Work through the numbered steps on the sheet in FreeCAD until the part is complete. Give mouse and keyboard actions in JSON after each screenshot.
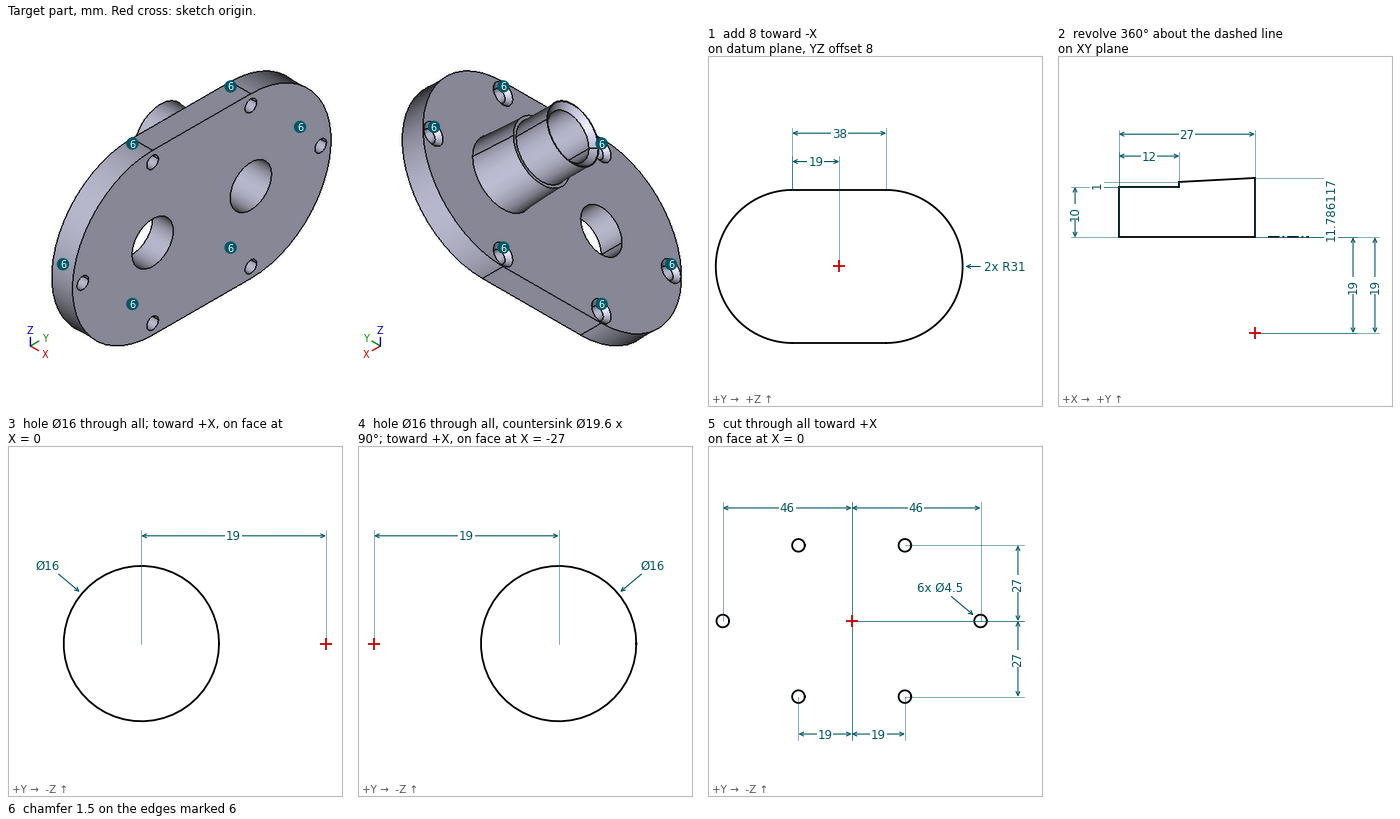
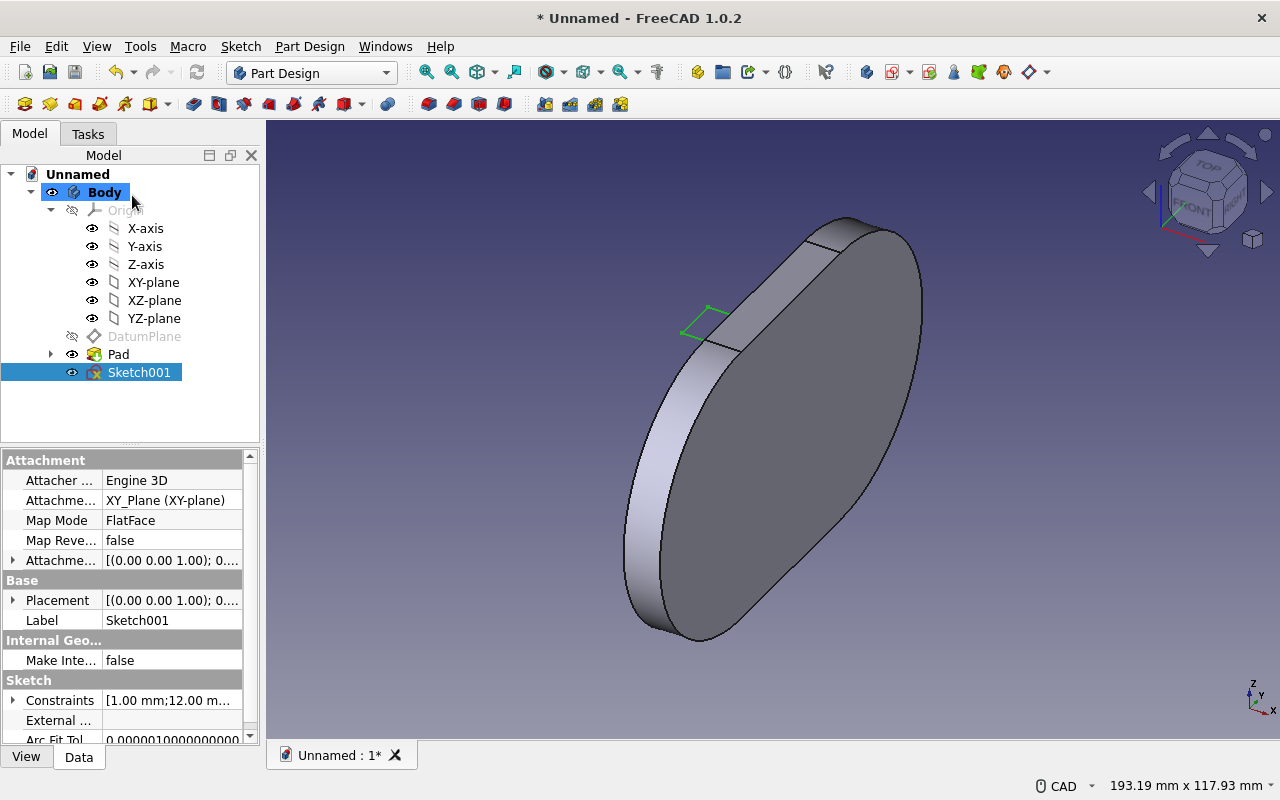
{"action": "left_click", "coordinate": [50, 104]}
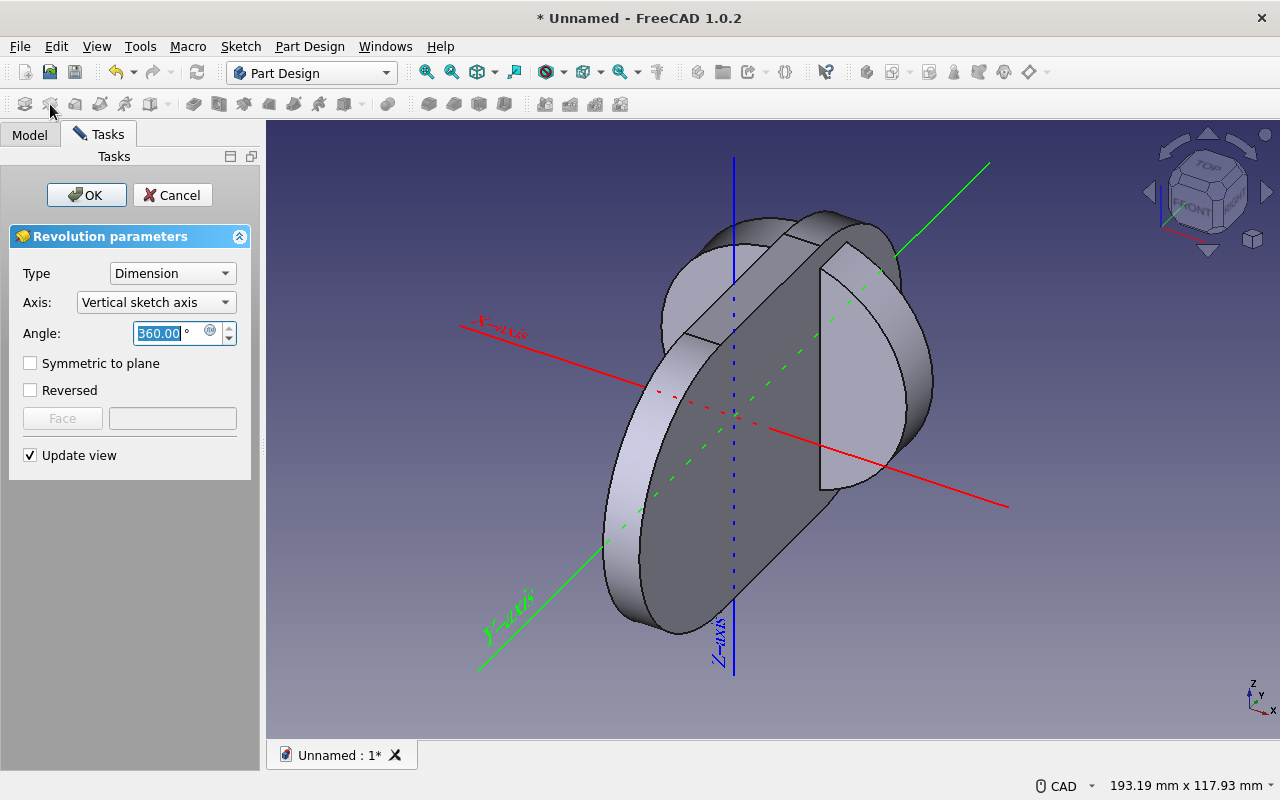
{"action": "left_click", "coordinate": [157, 302]}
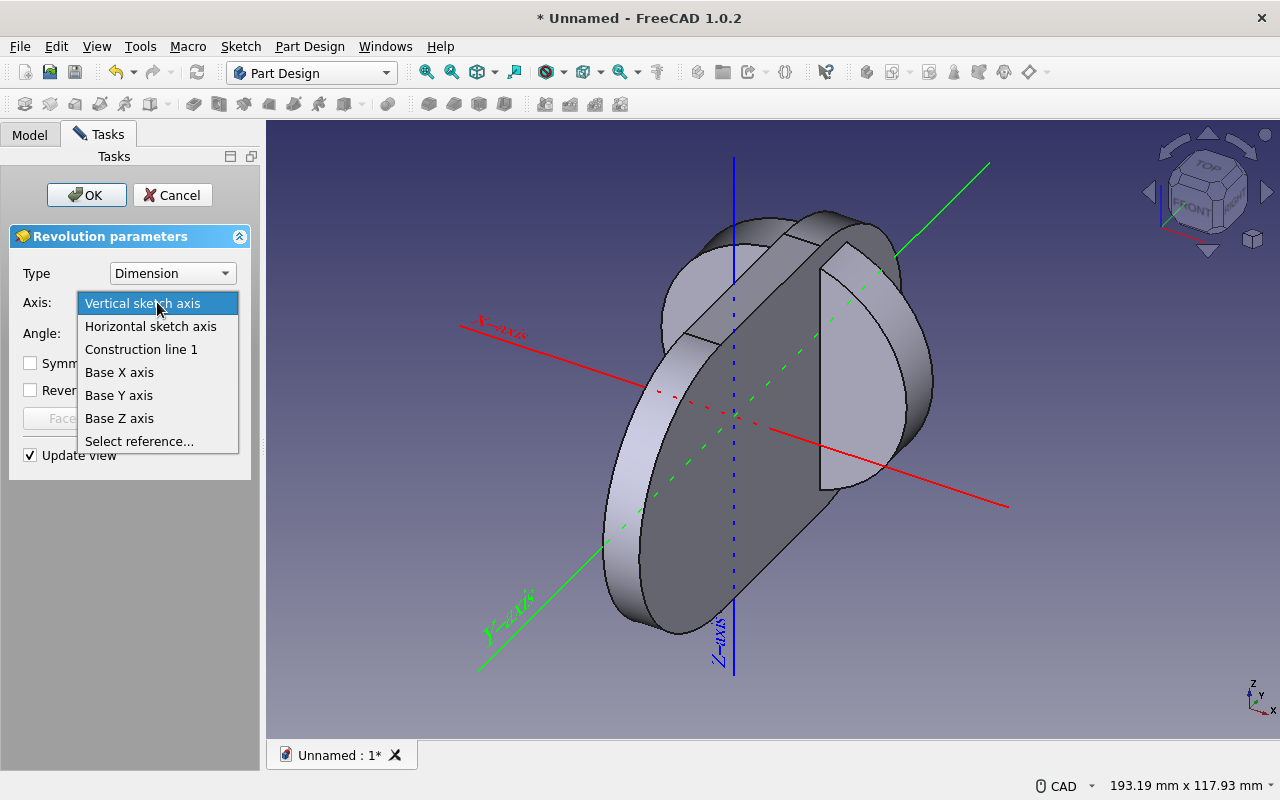
{"action": "left_click", "coordinate": [156, 350]}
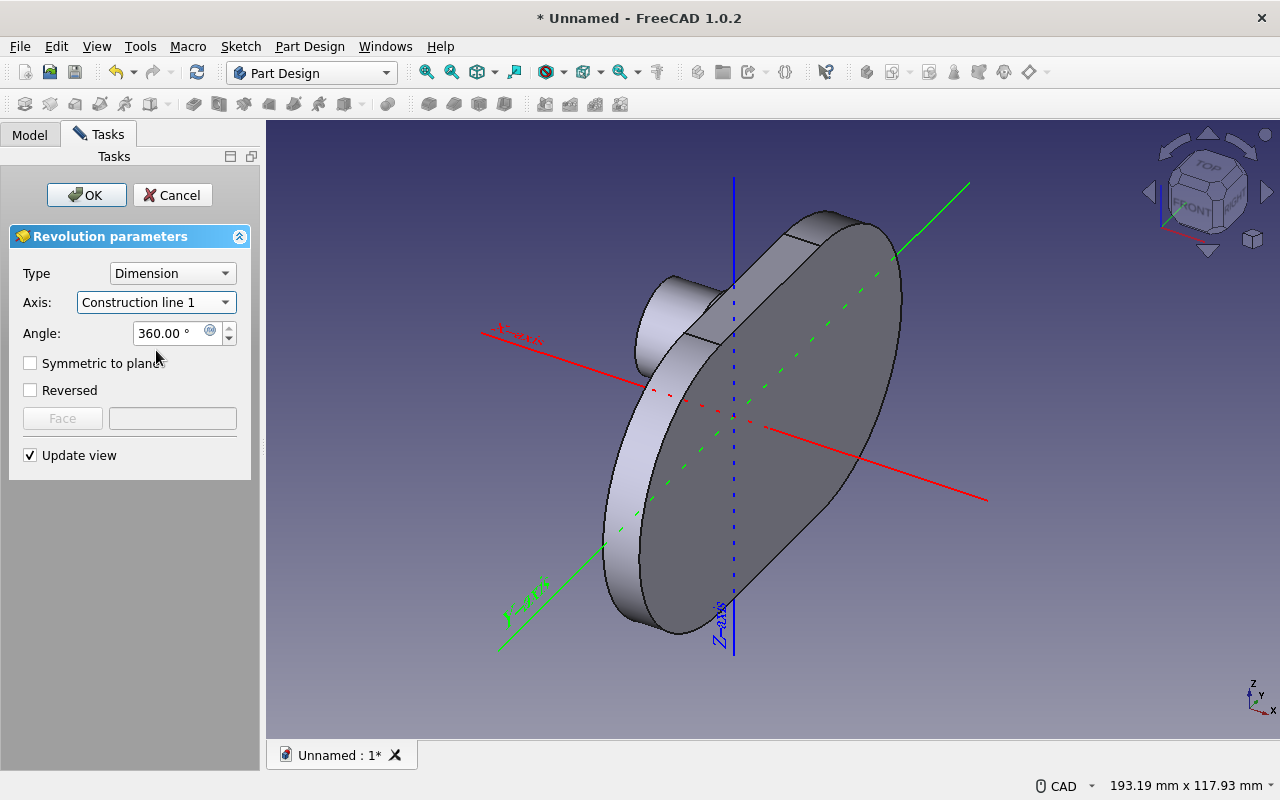
{"action": "left_click", "coordinate": [87, 195]}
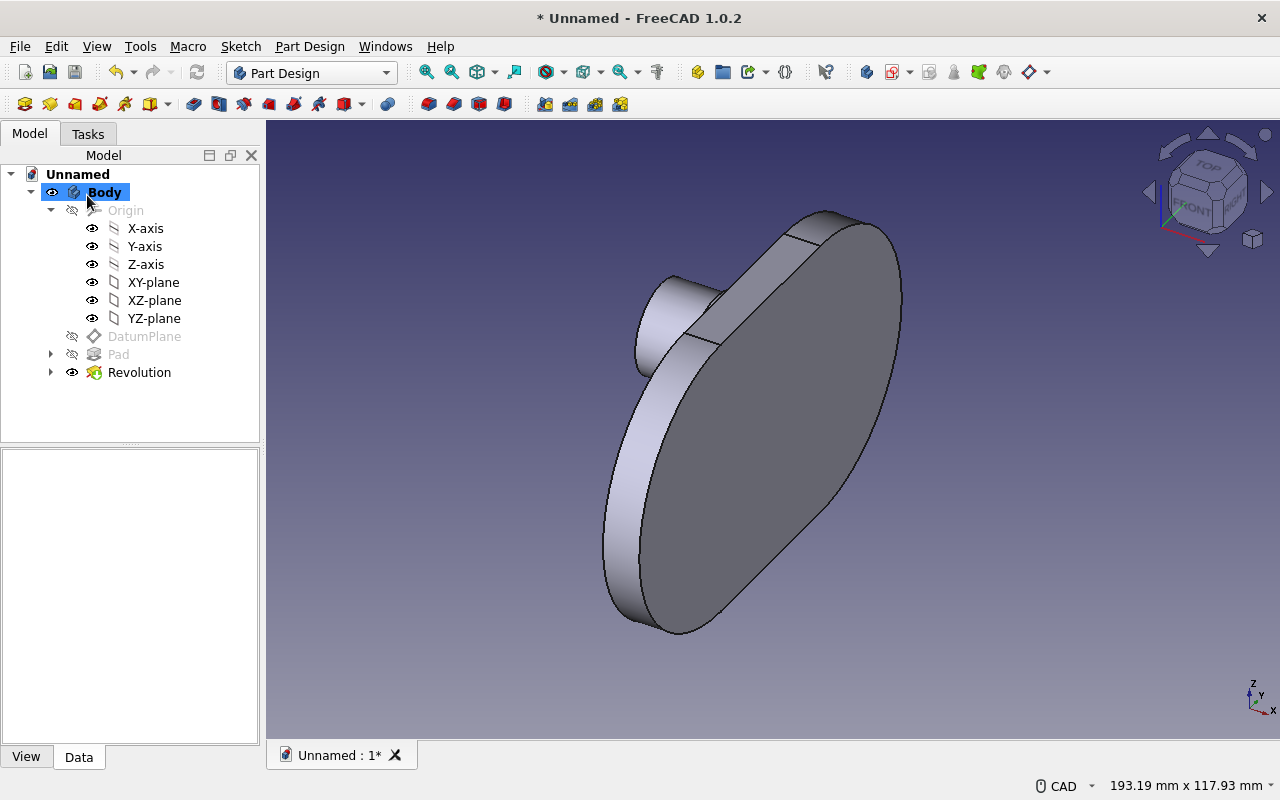
{"action": "left_click", "coordinate": [427, 72]}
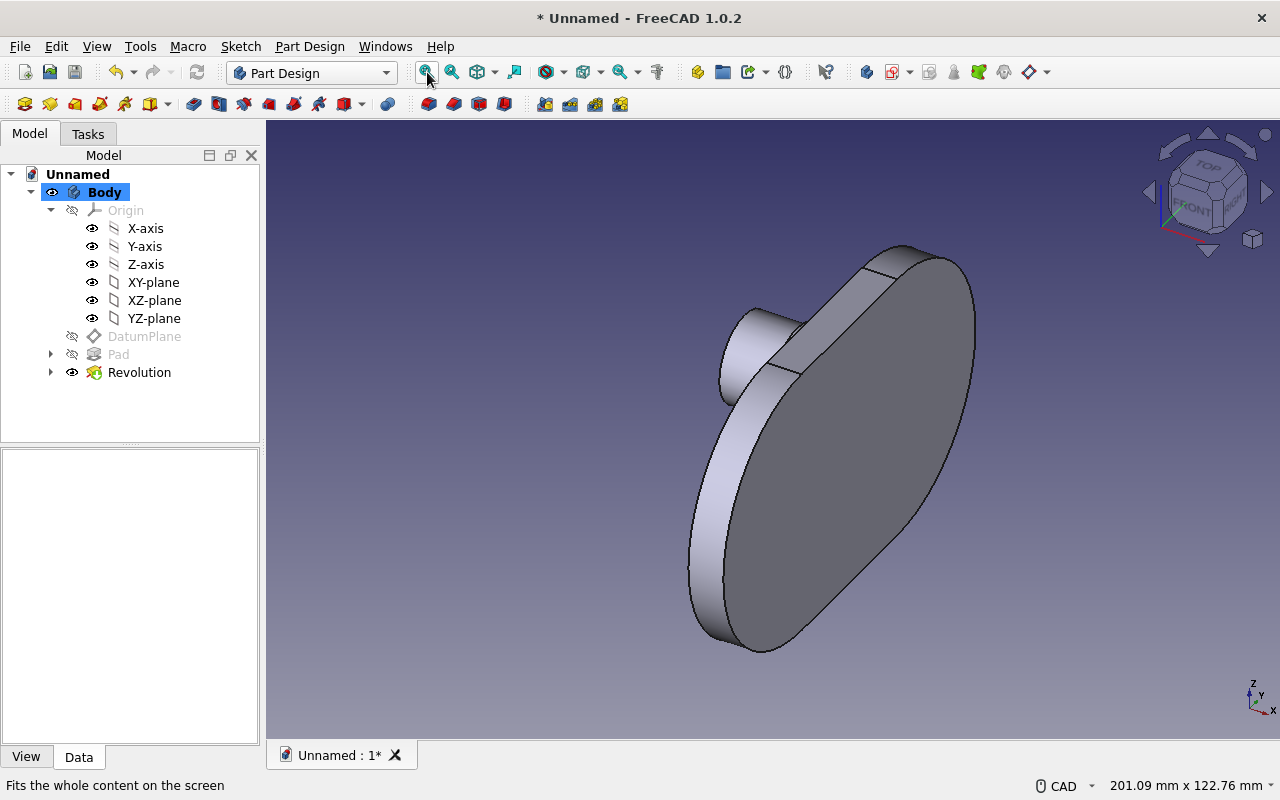
{"action": "key", "text": "6"}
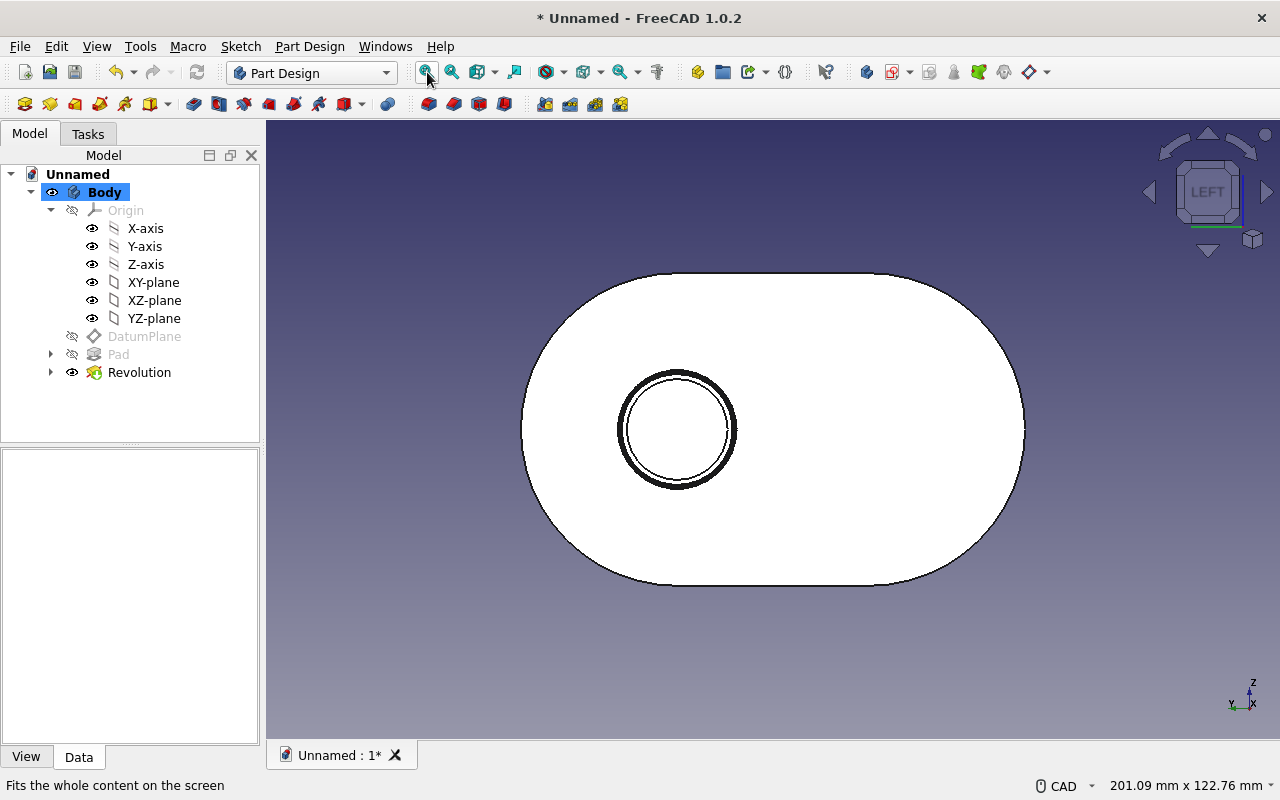
{"action": "left_click", "coordinate": [845, 384]}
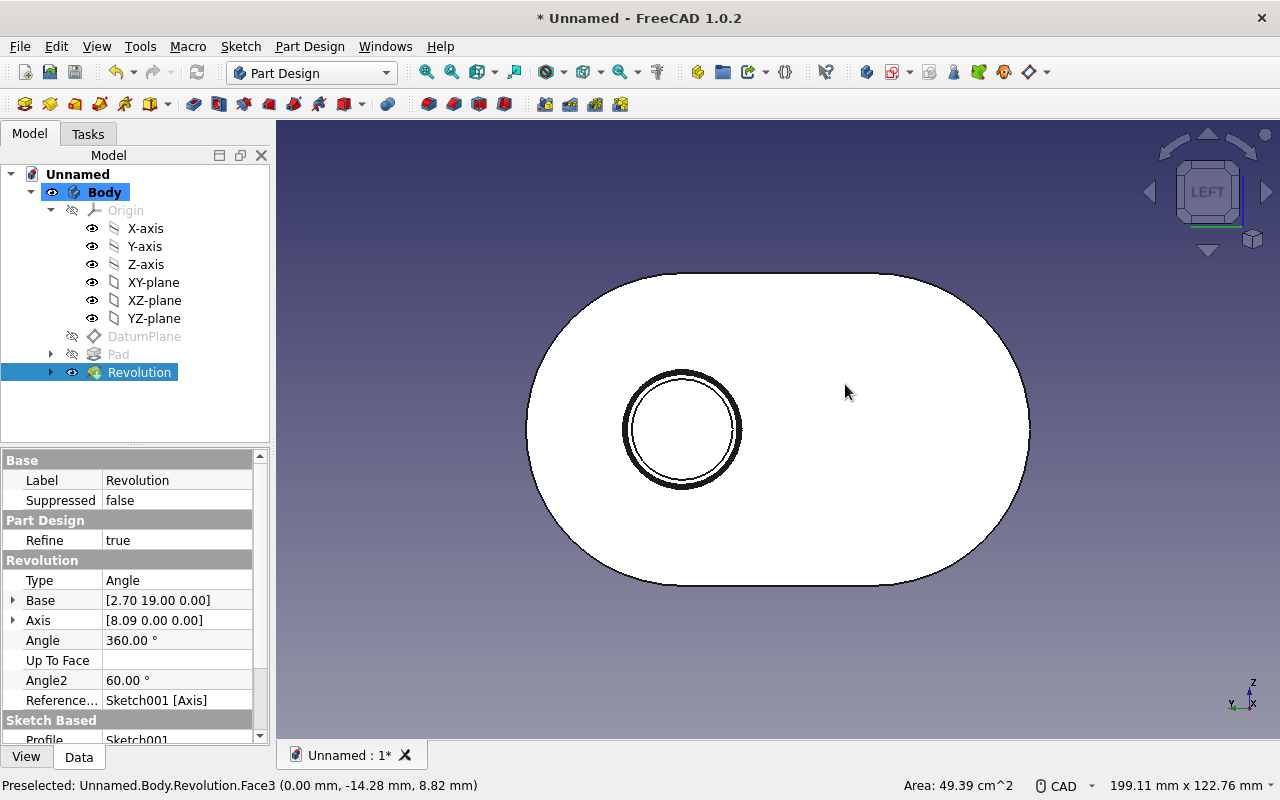
{"action": "left_click", "coordinate": [892, 72]}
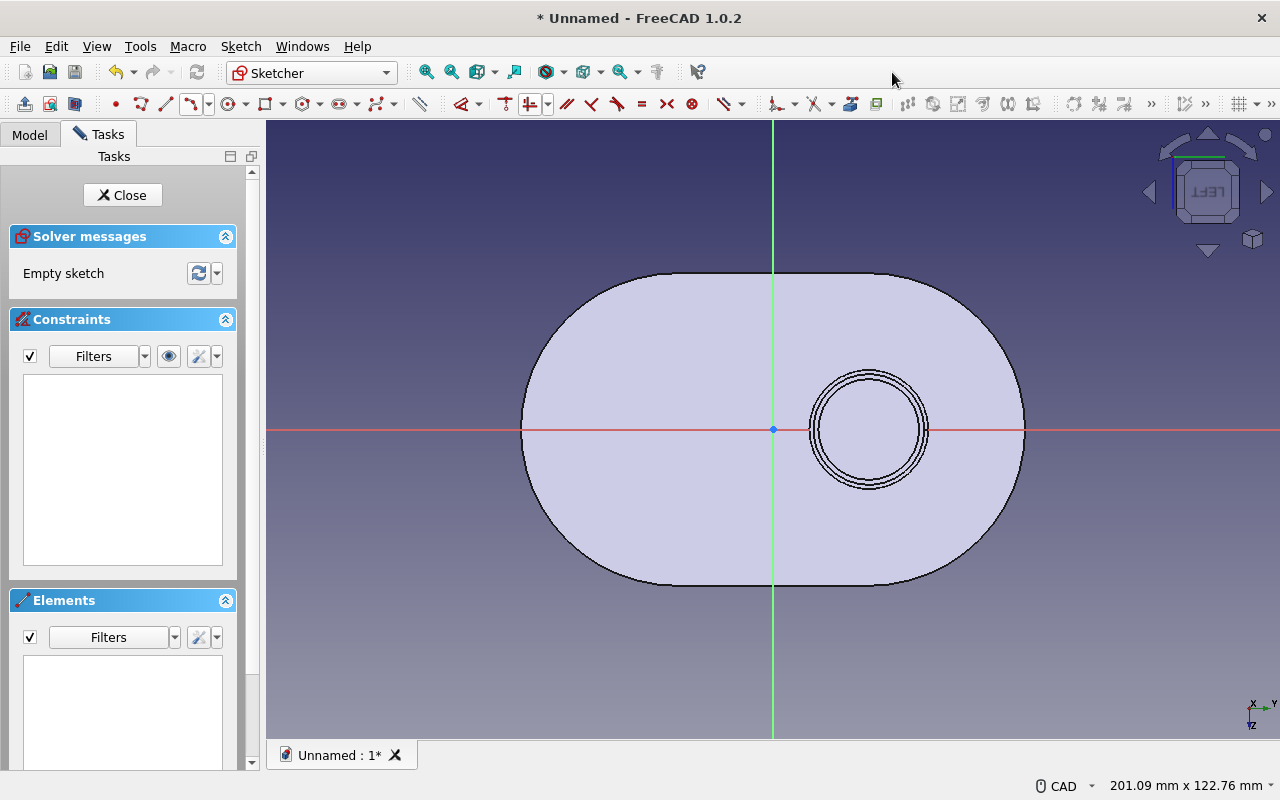
{"action": "left_click", "coordinate": [75, 104]}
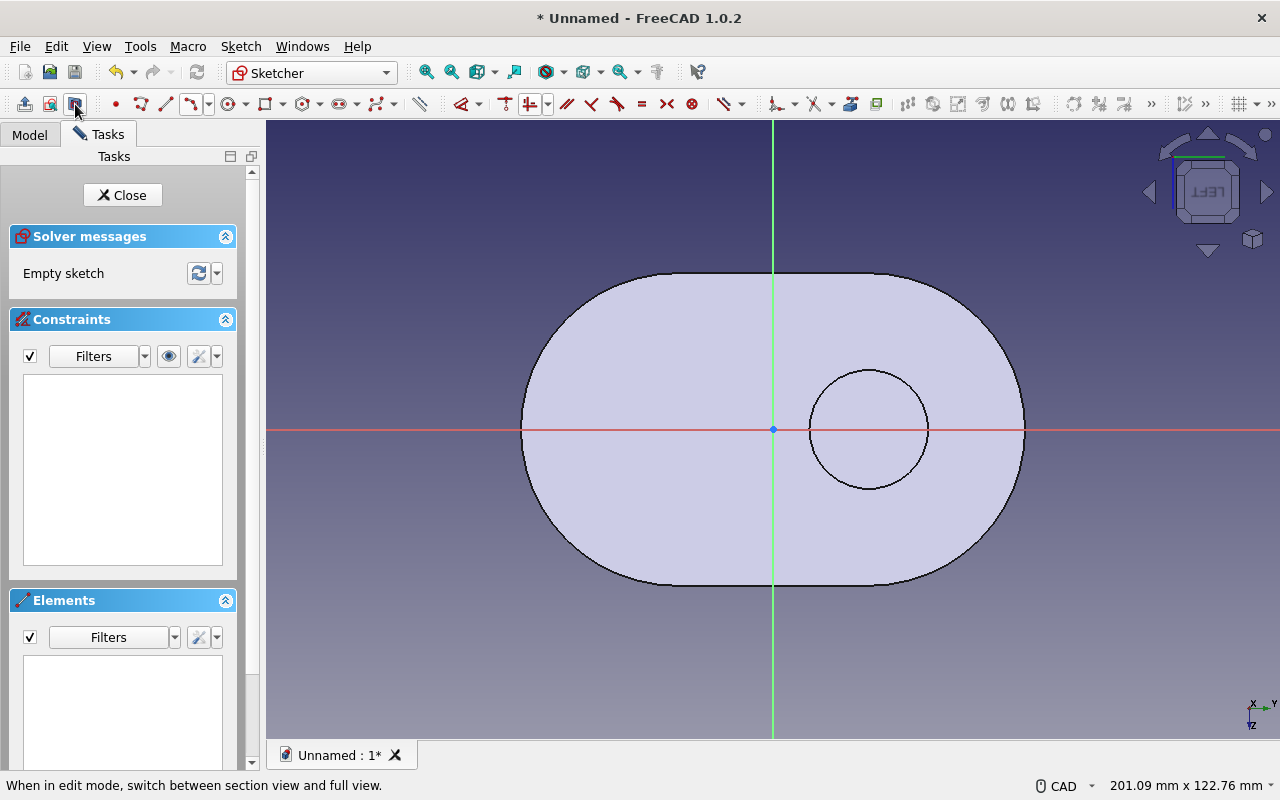
{"action": "scroll", "coordinate": [705, 430], "scroll_direction": "up", "scroll_amount": 7}